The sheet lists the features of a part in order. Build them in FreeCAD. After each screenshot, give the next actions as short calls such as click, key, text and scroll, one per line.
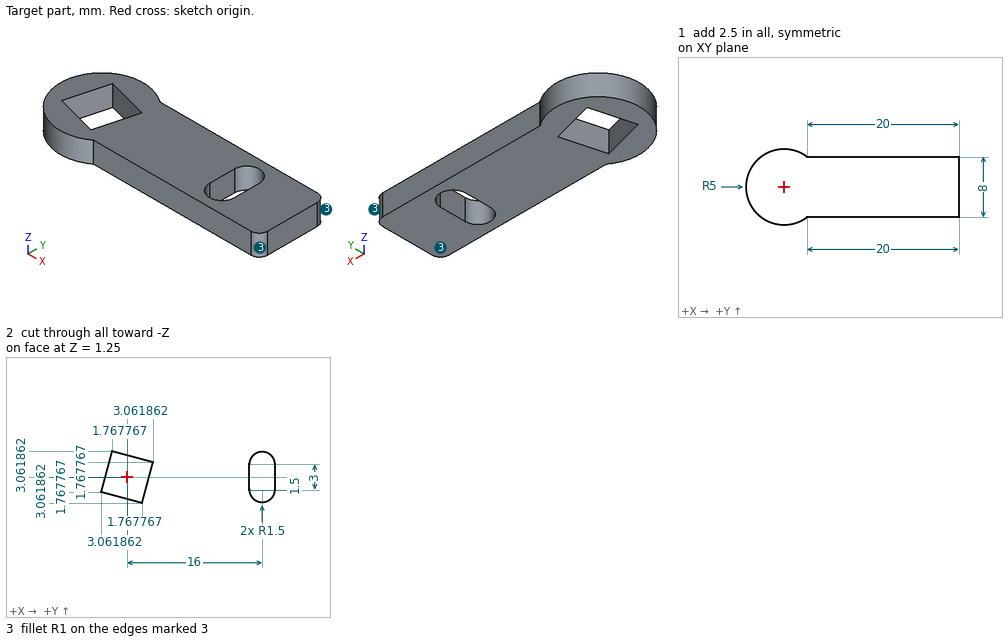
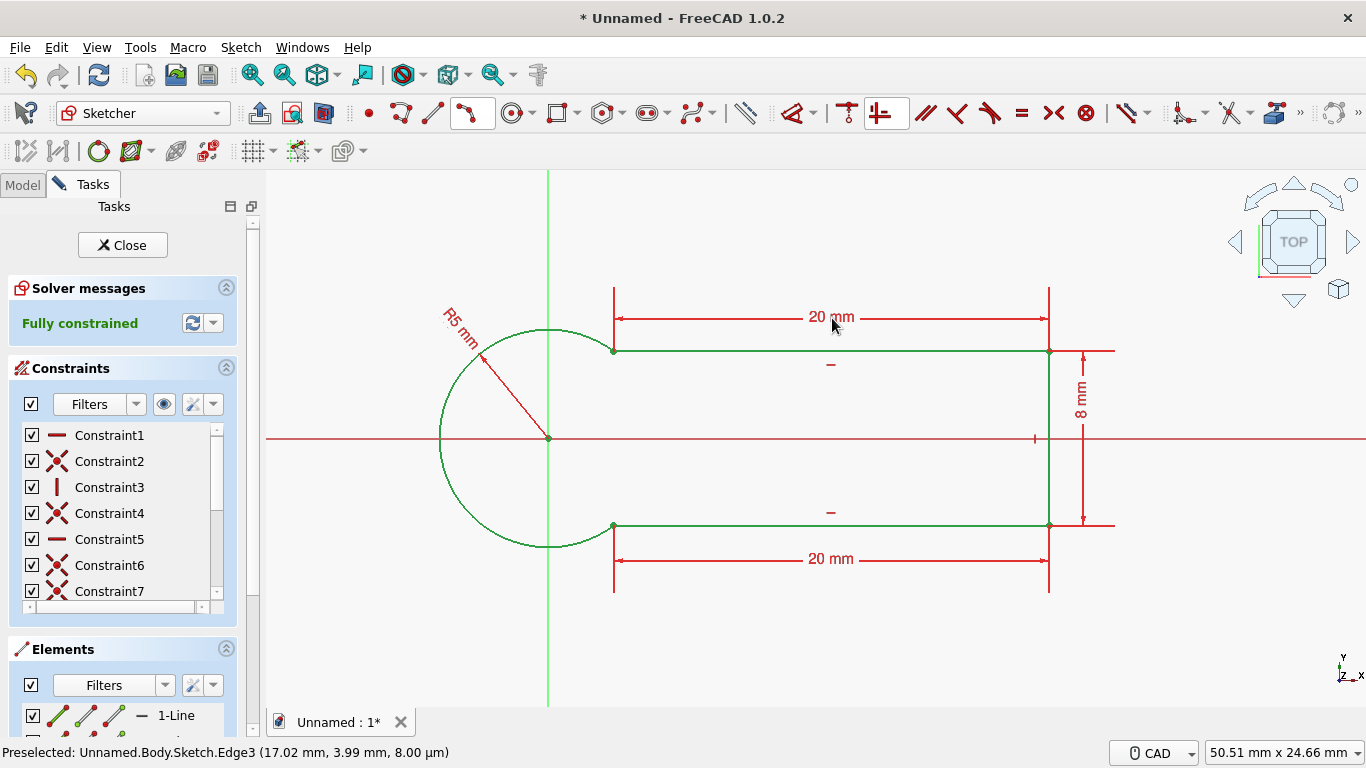
click(123, 245)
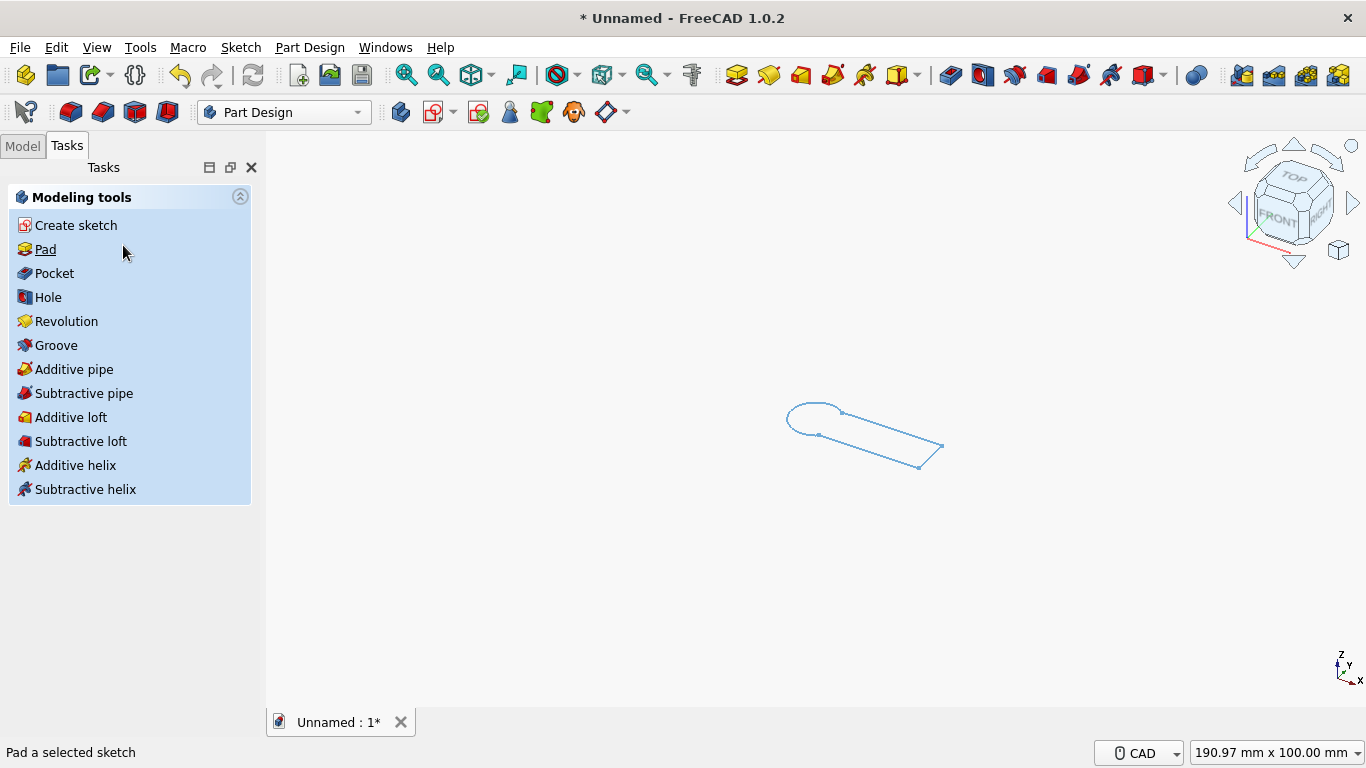
click(738, 76)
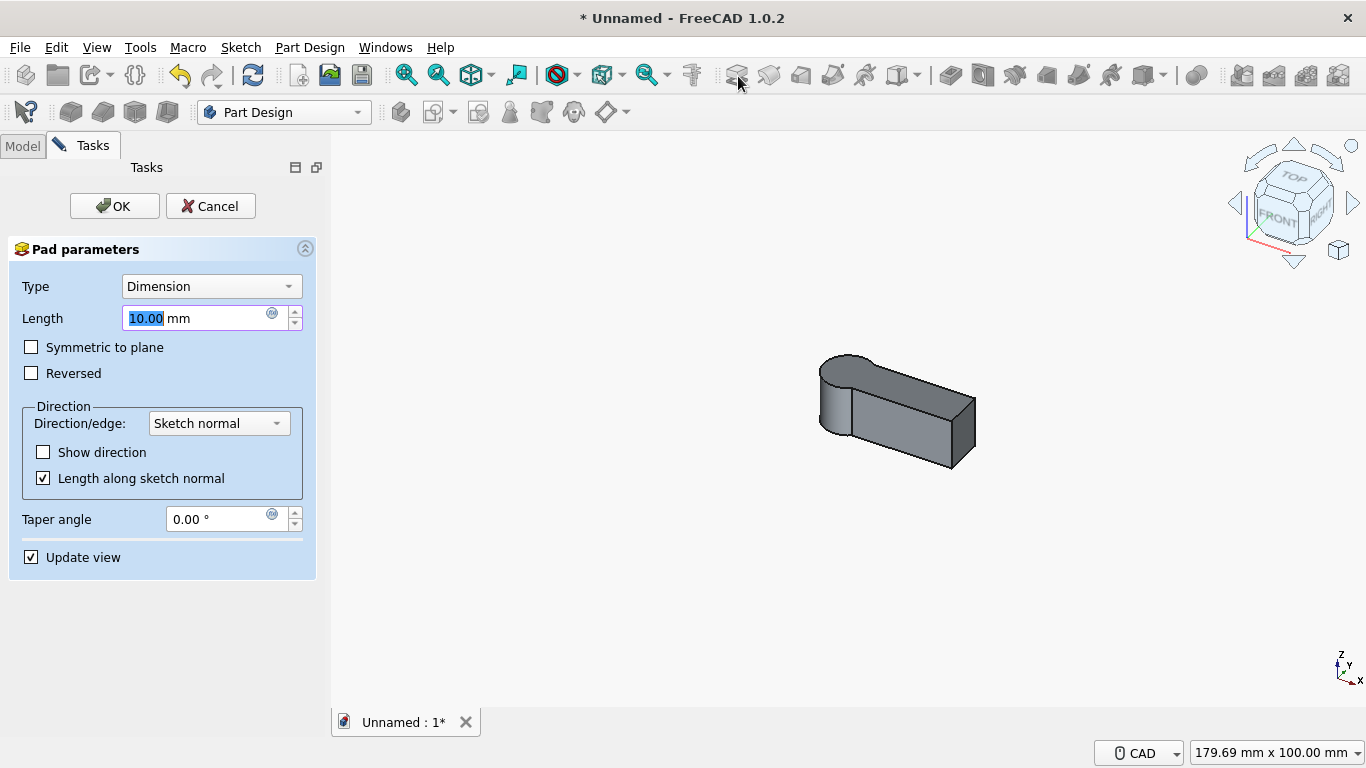
text(2.5)
key(Tab)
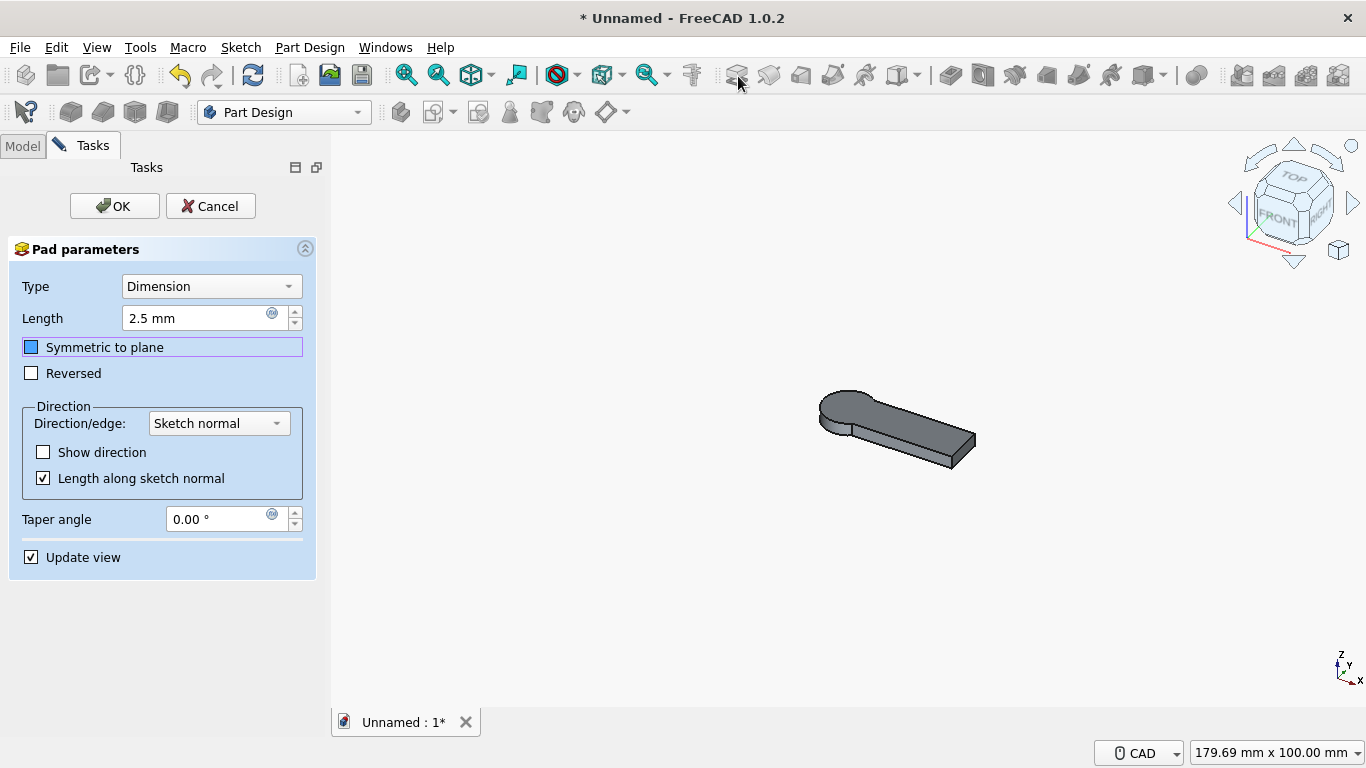
click(30, 347)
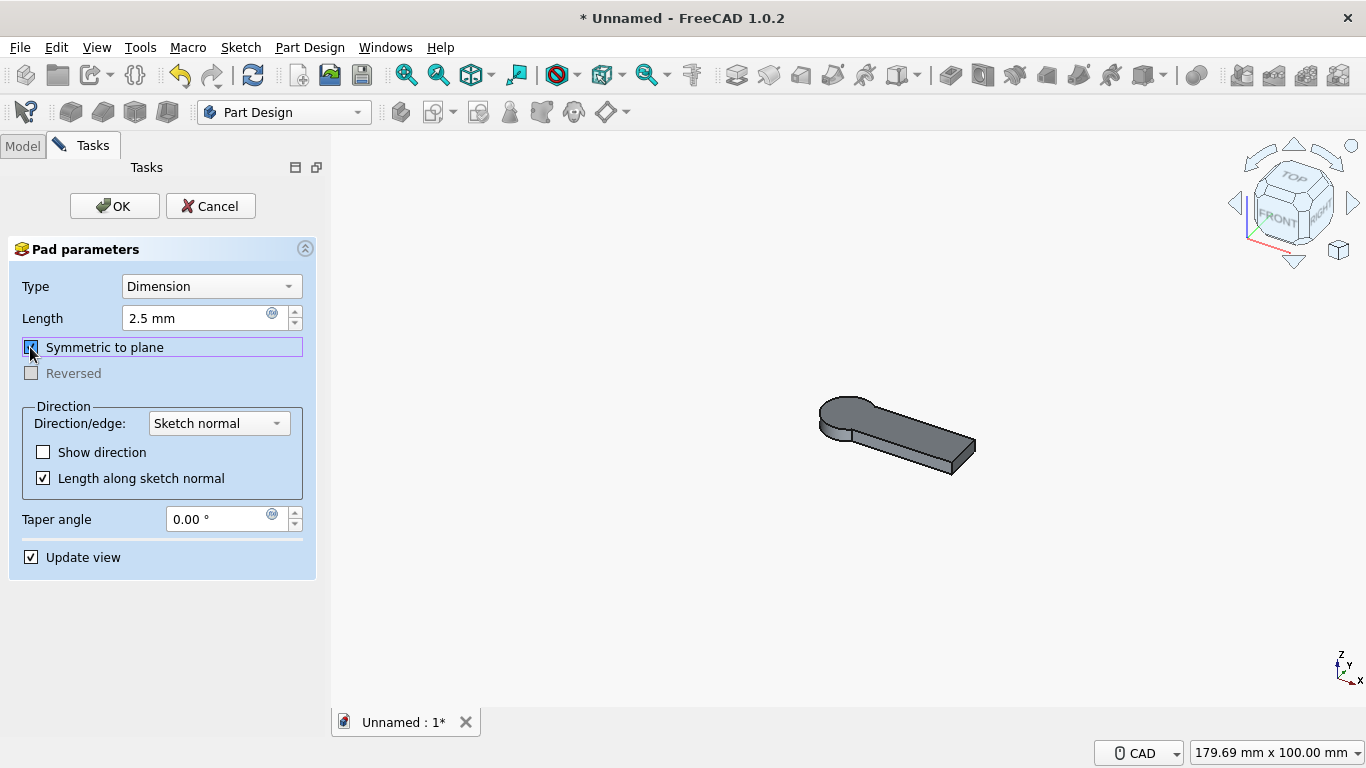
click(115, 206)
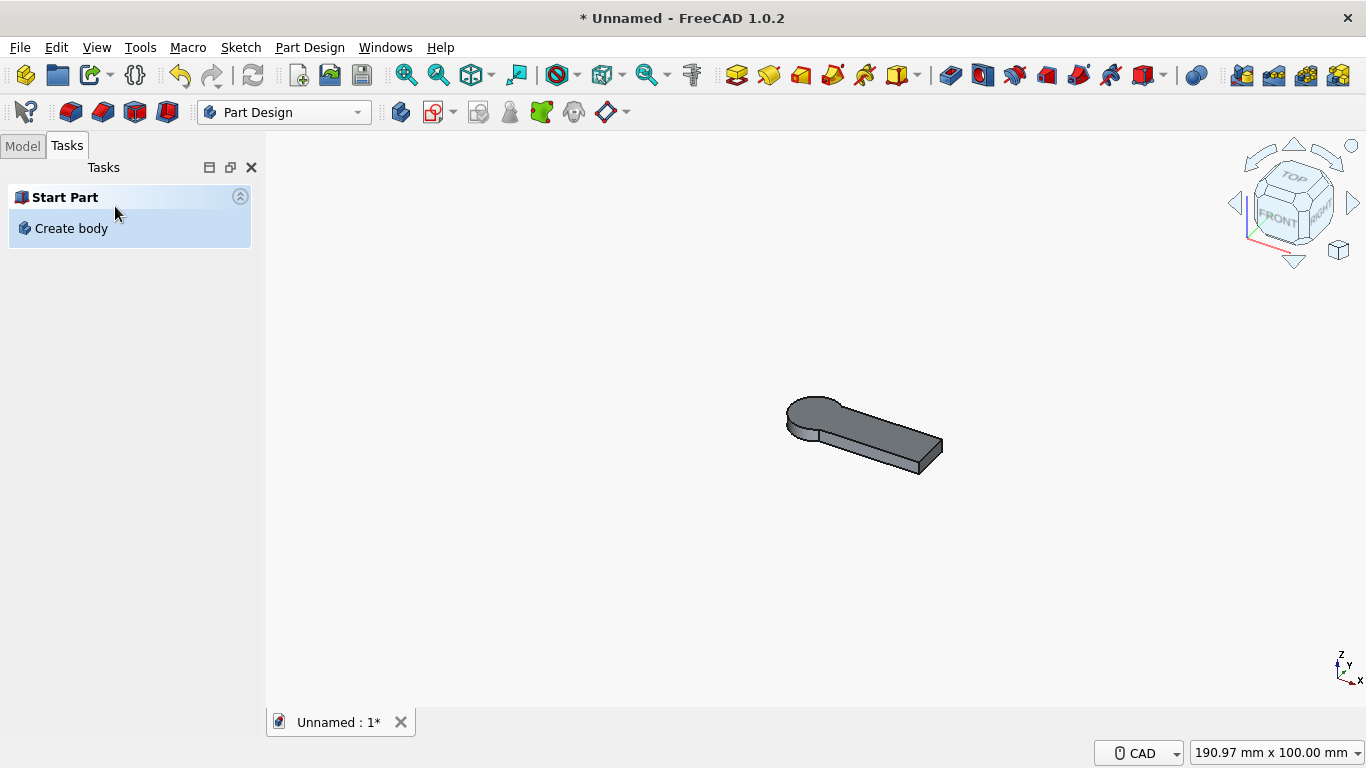
click(408, 76)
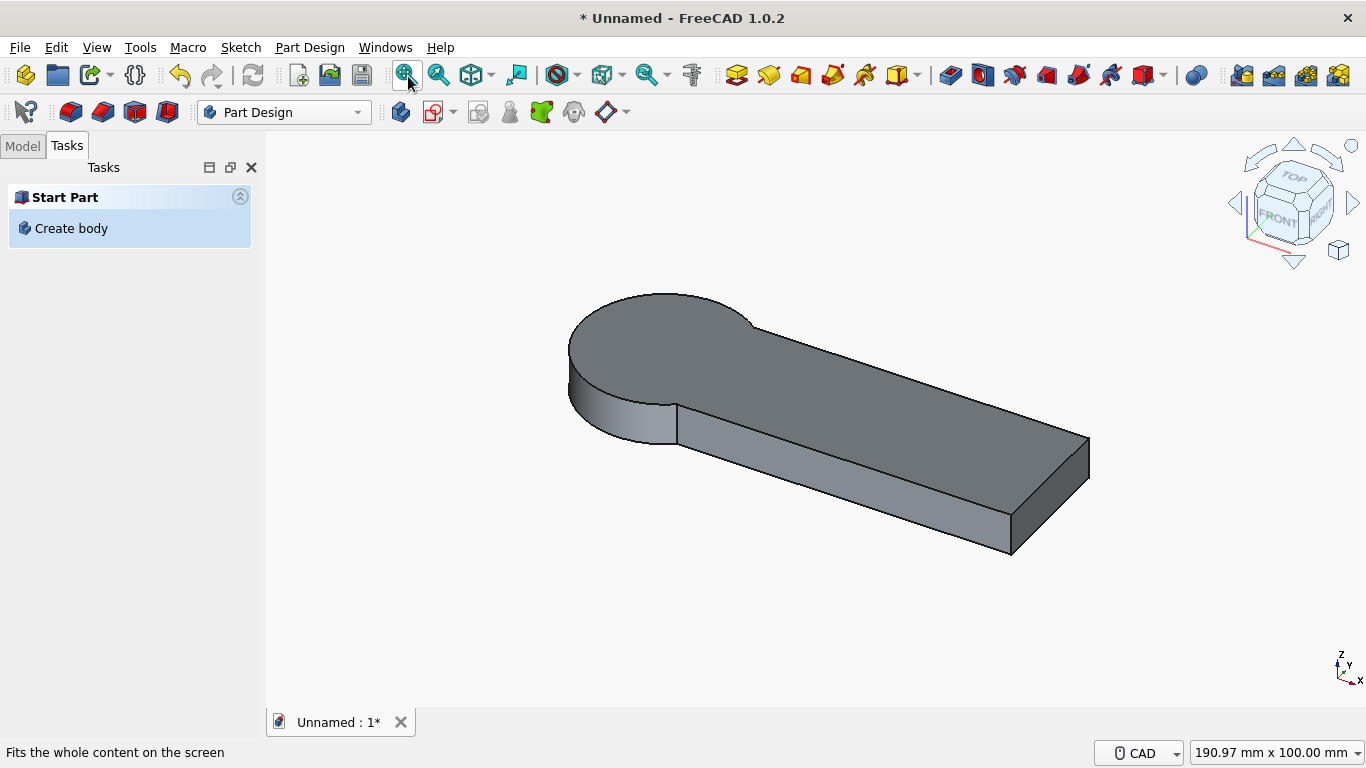
click(682, 354)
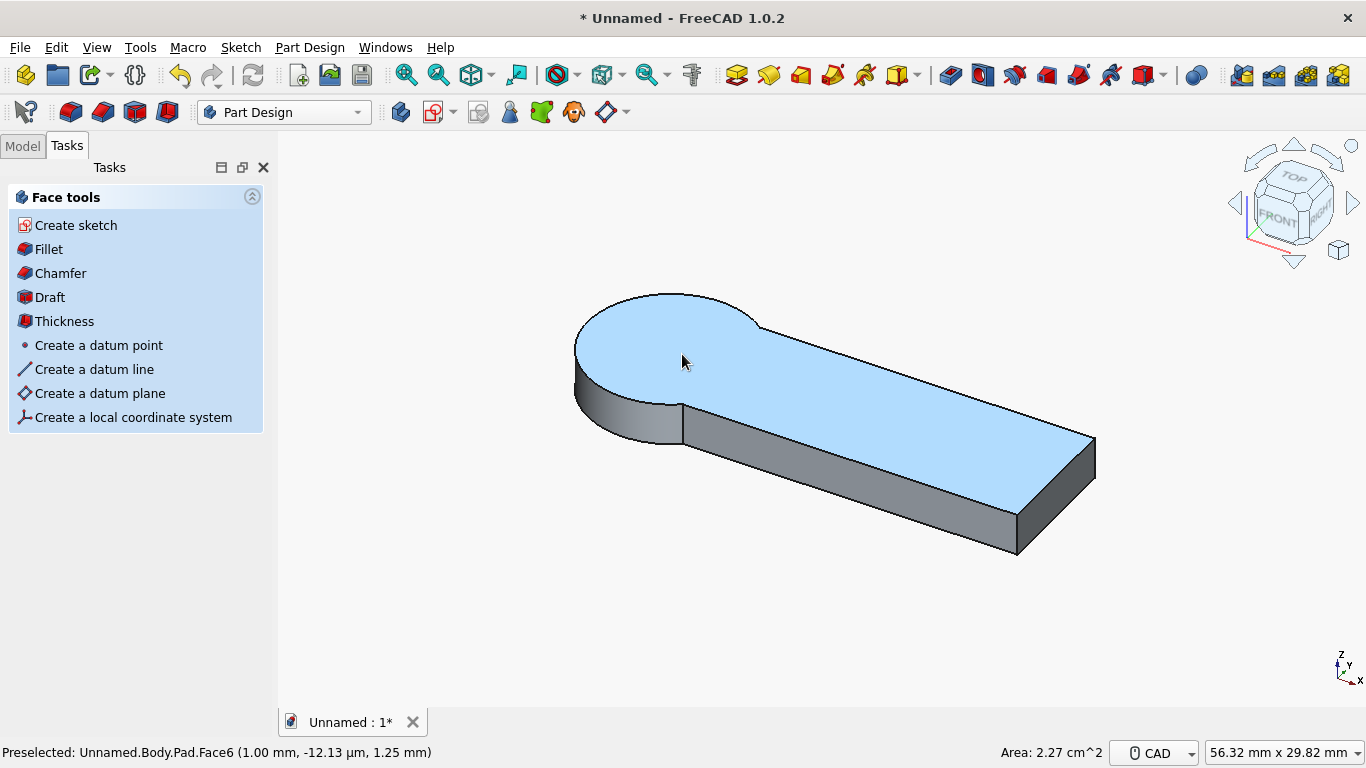
click(434, 112)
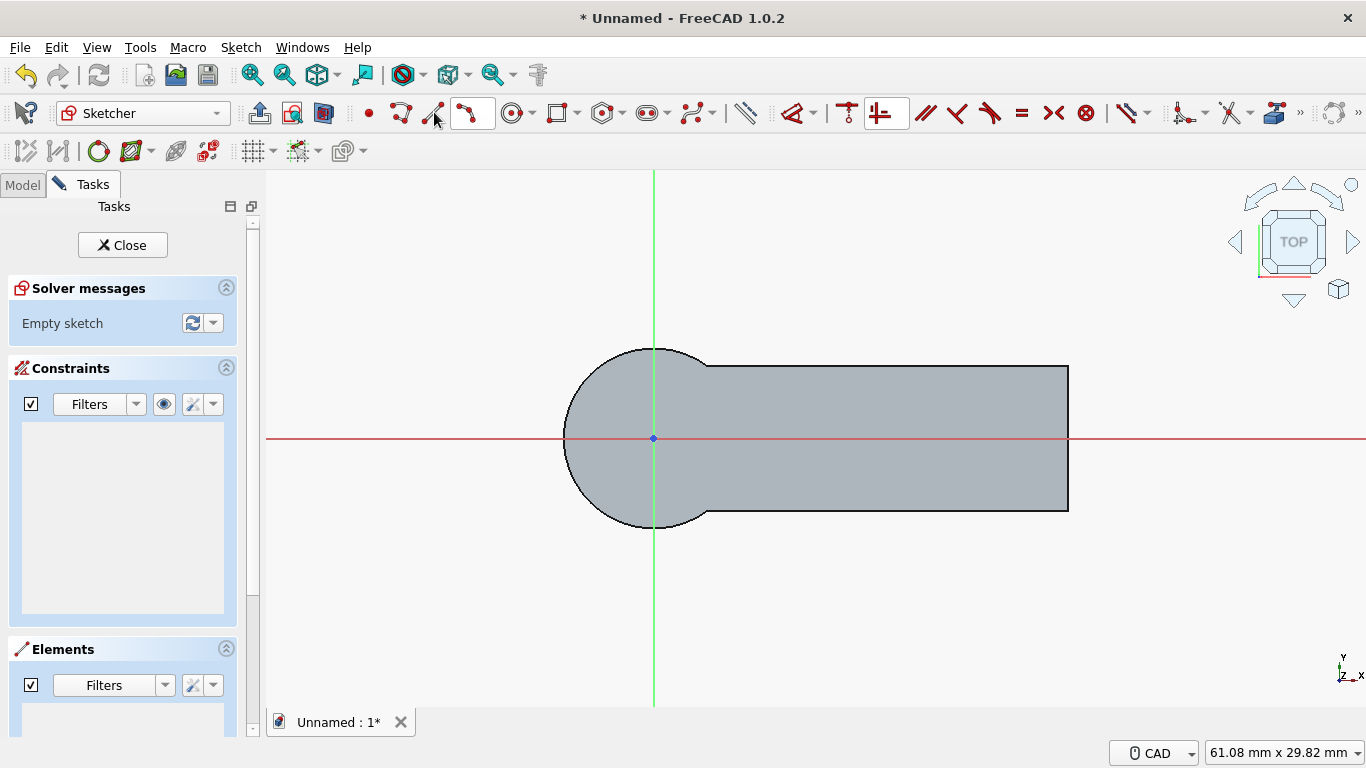
scroll(828, 438, up, 3)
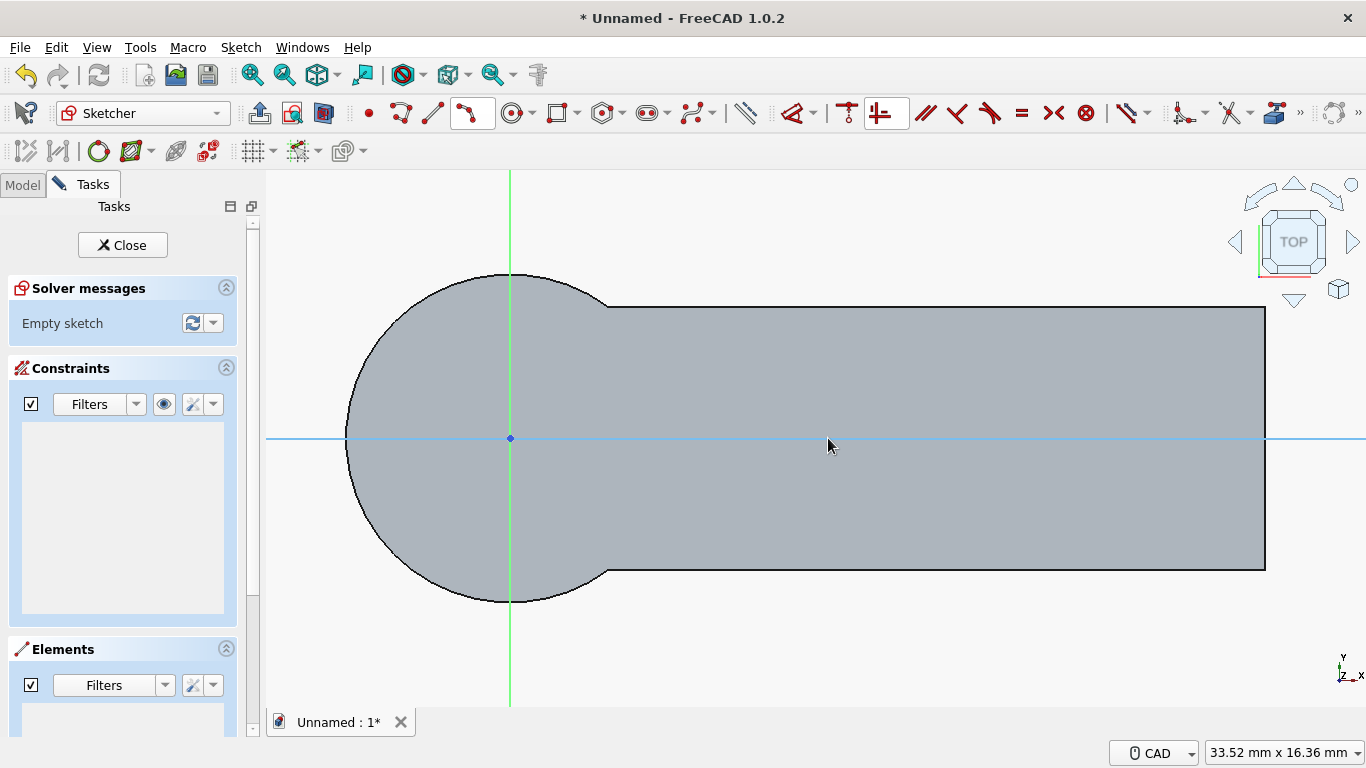
click(402, 114)